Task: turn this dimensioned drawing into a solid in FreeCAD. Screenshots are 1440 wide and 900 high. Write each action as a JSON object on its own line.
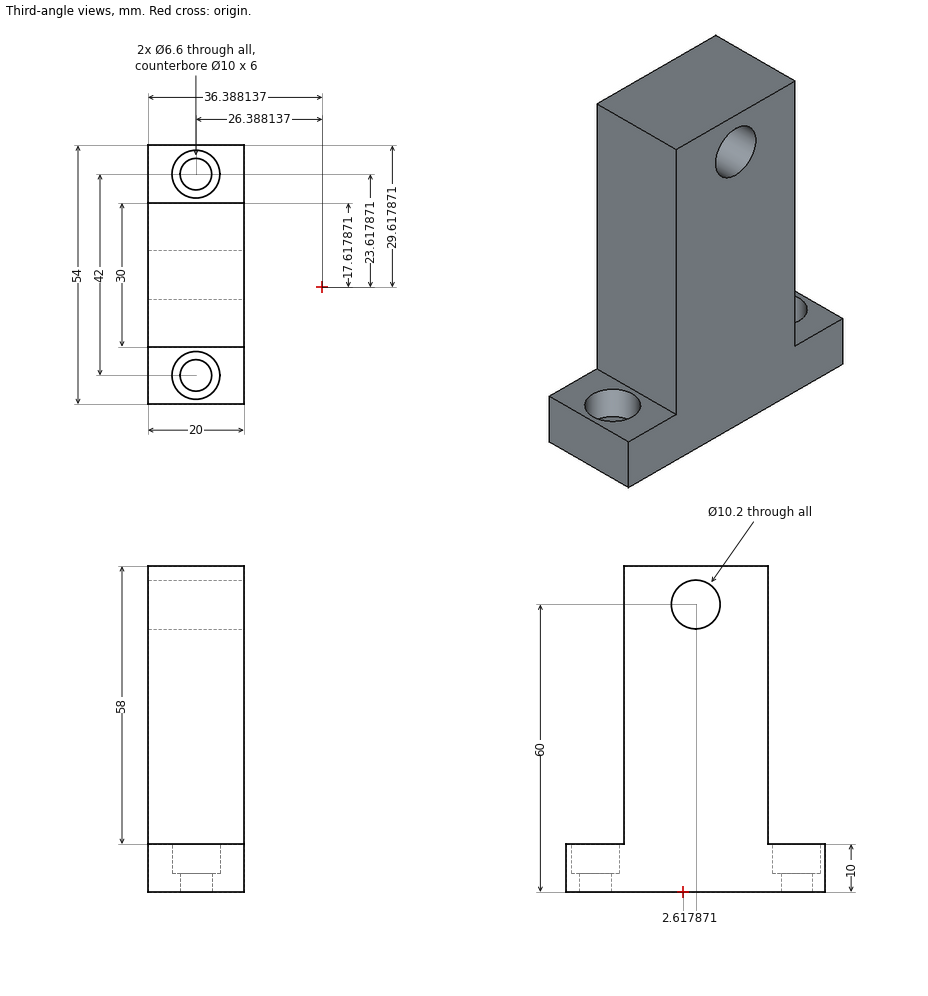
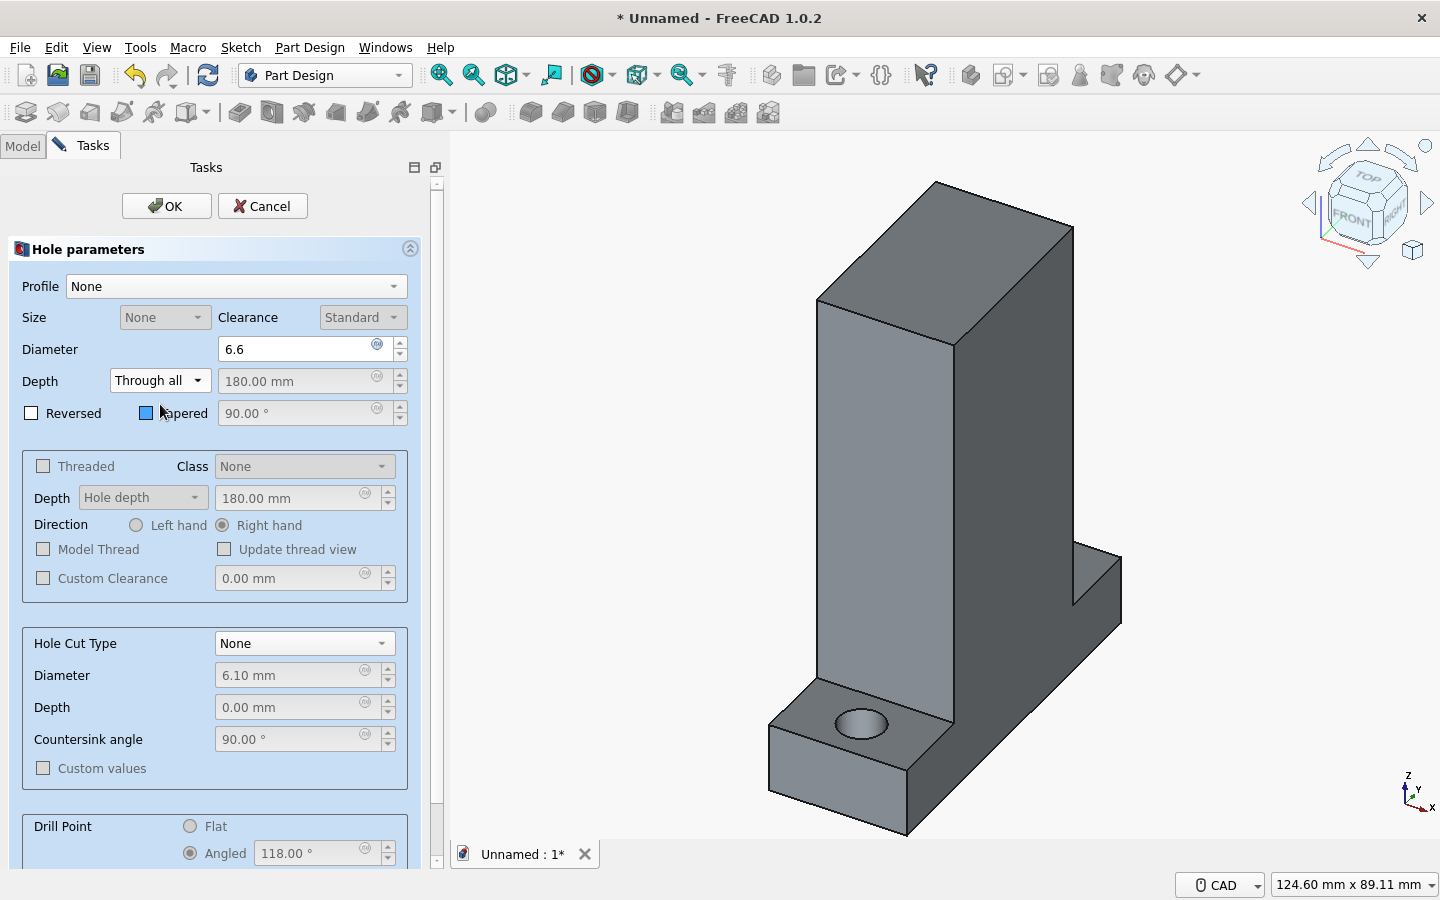
{"action": "left_click", "coordinate": [306, 644]}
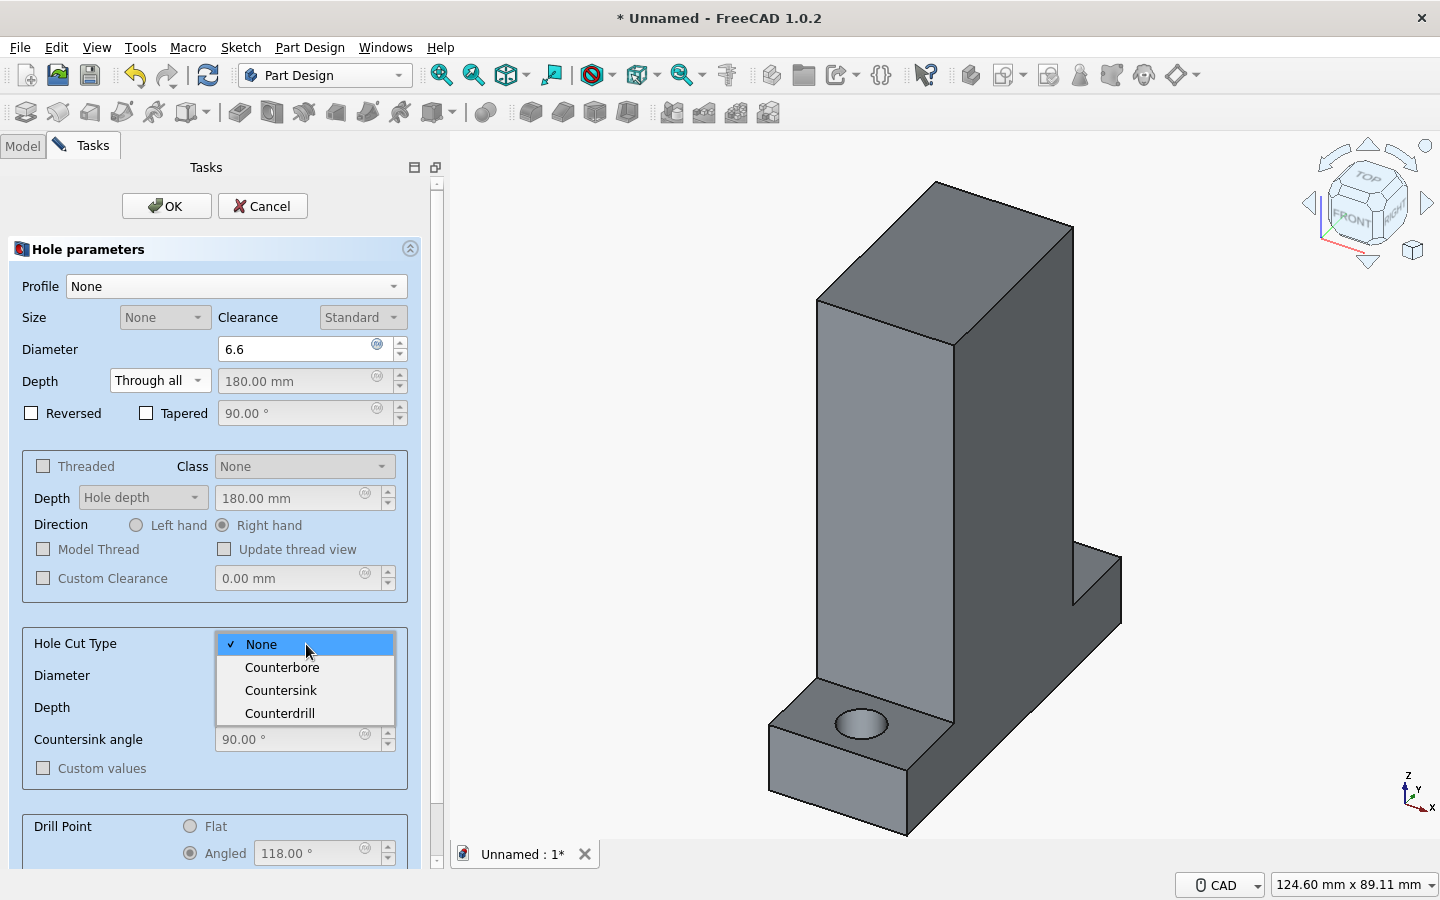
{"action": "left_click", "coordinate": [304, 668]}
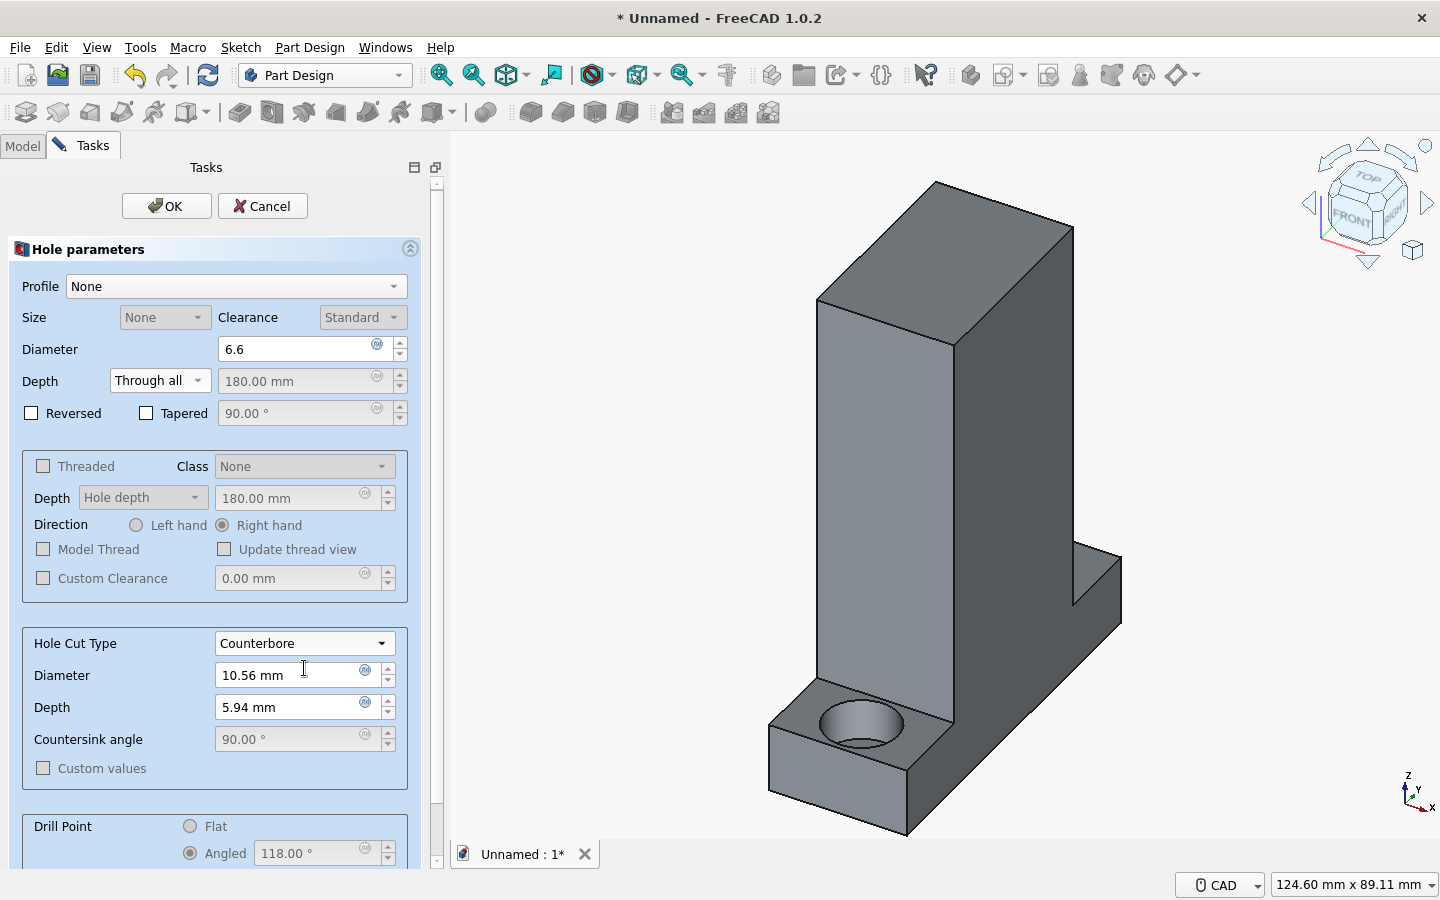
{"action": "triple_click", "coordinate": [298, 675]}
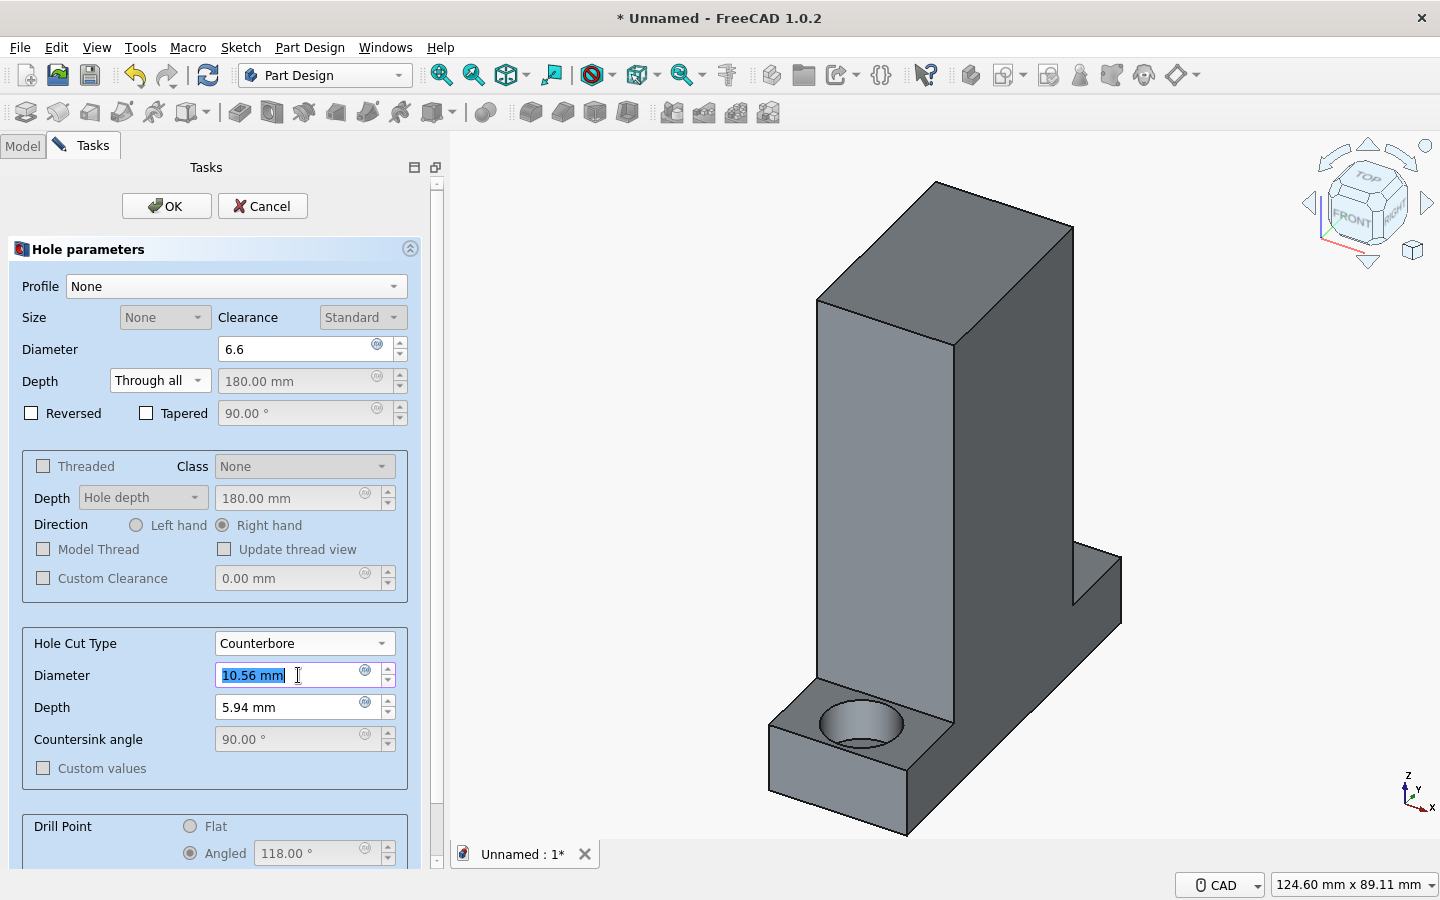
{"action": "type", "text": "10"}
{"action": "key", "text": "Tab"}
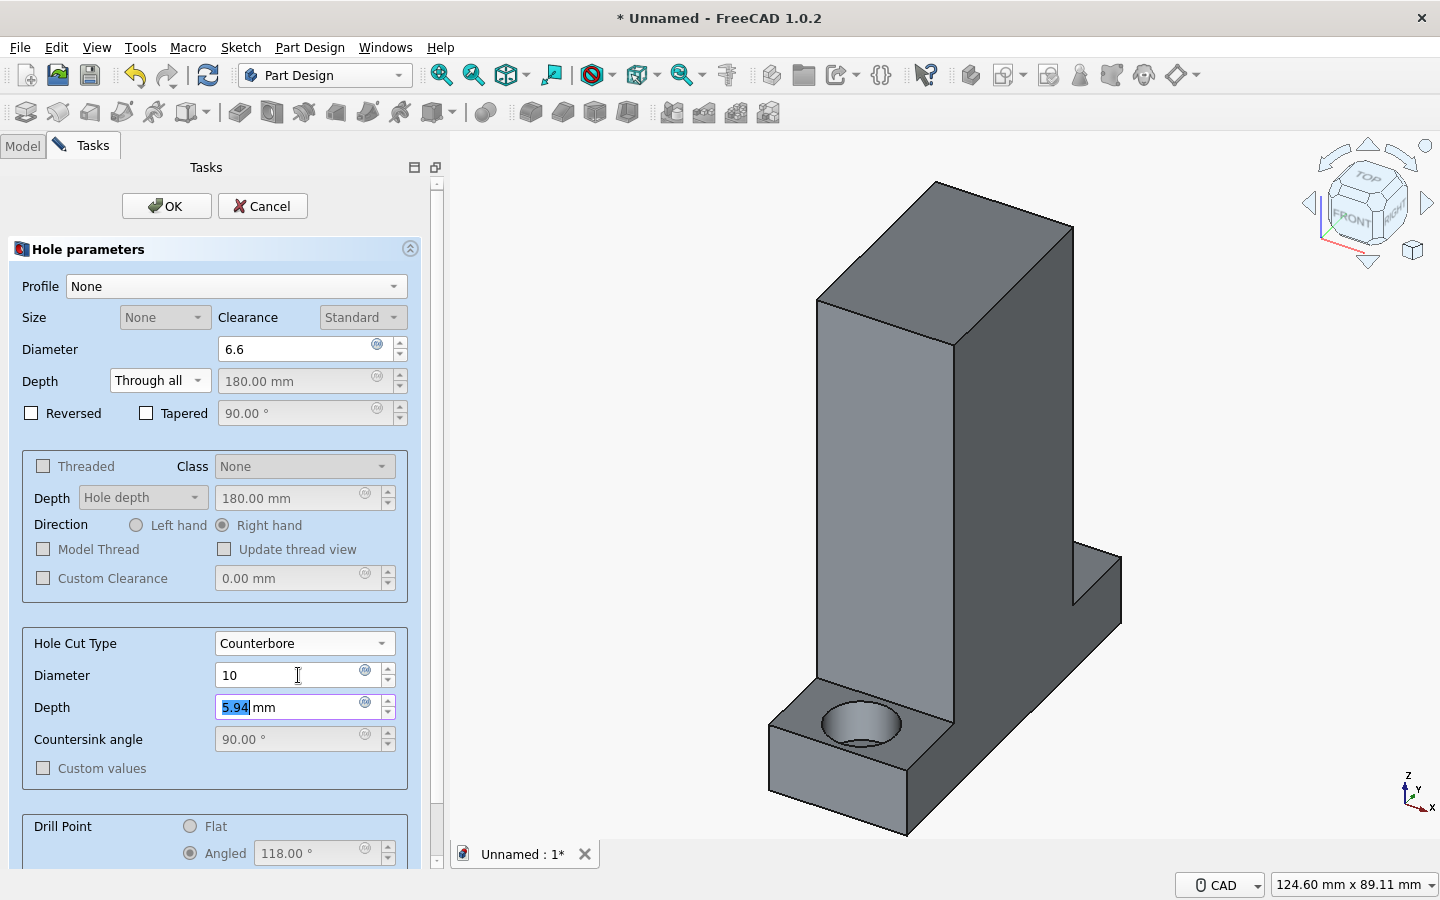
{"action": "type", "text": "6"}
{"action": "key", "text": "Tab"}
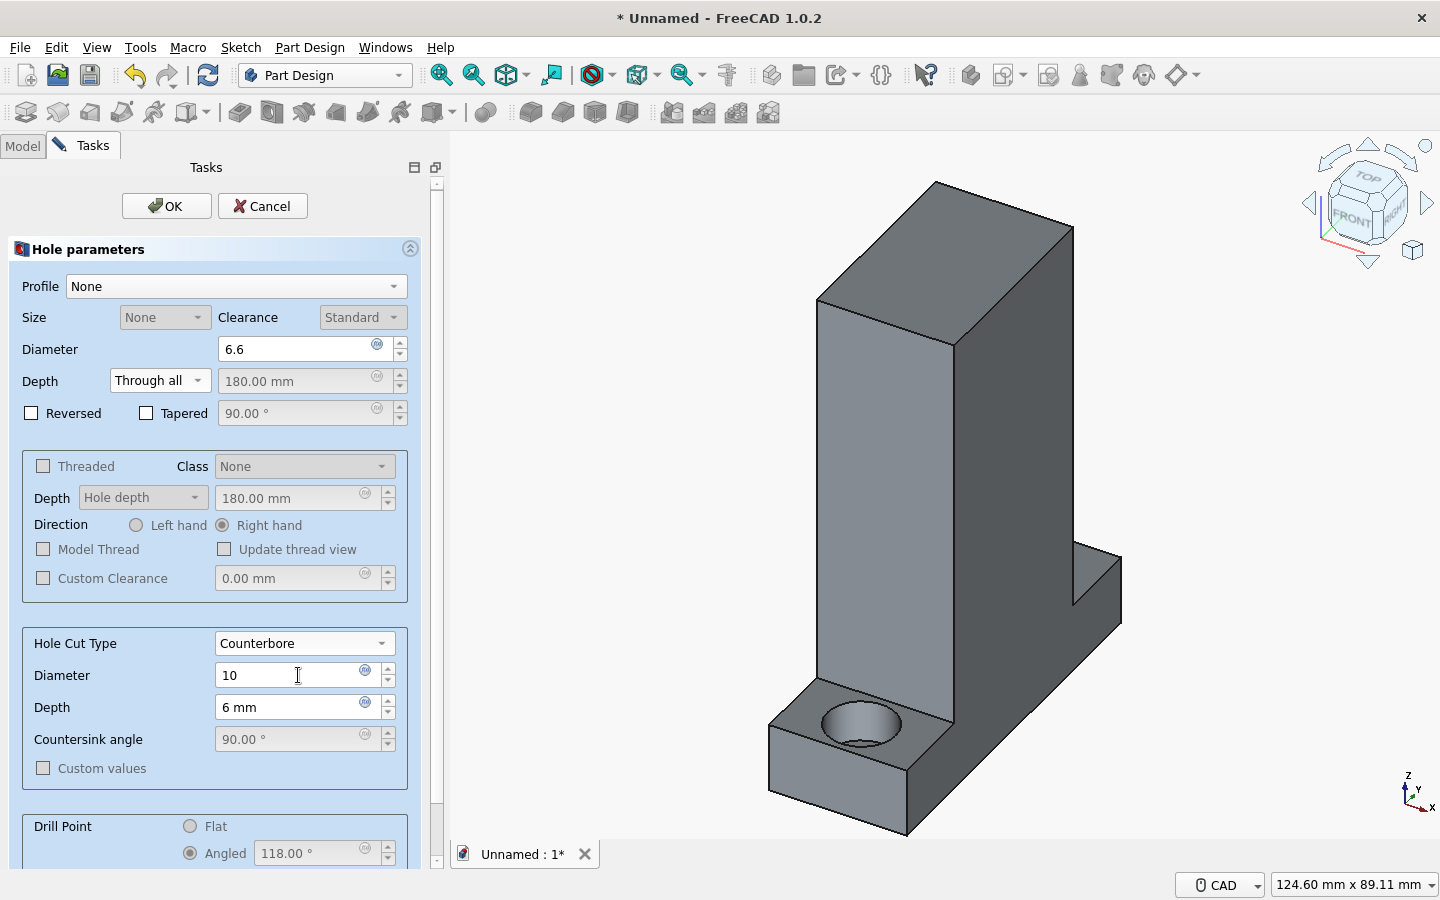
{"action": "left_click", "coordinate": [167, 206]}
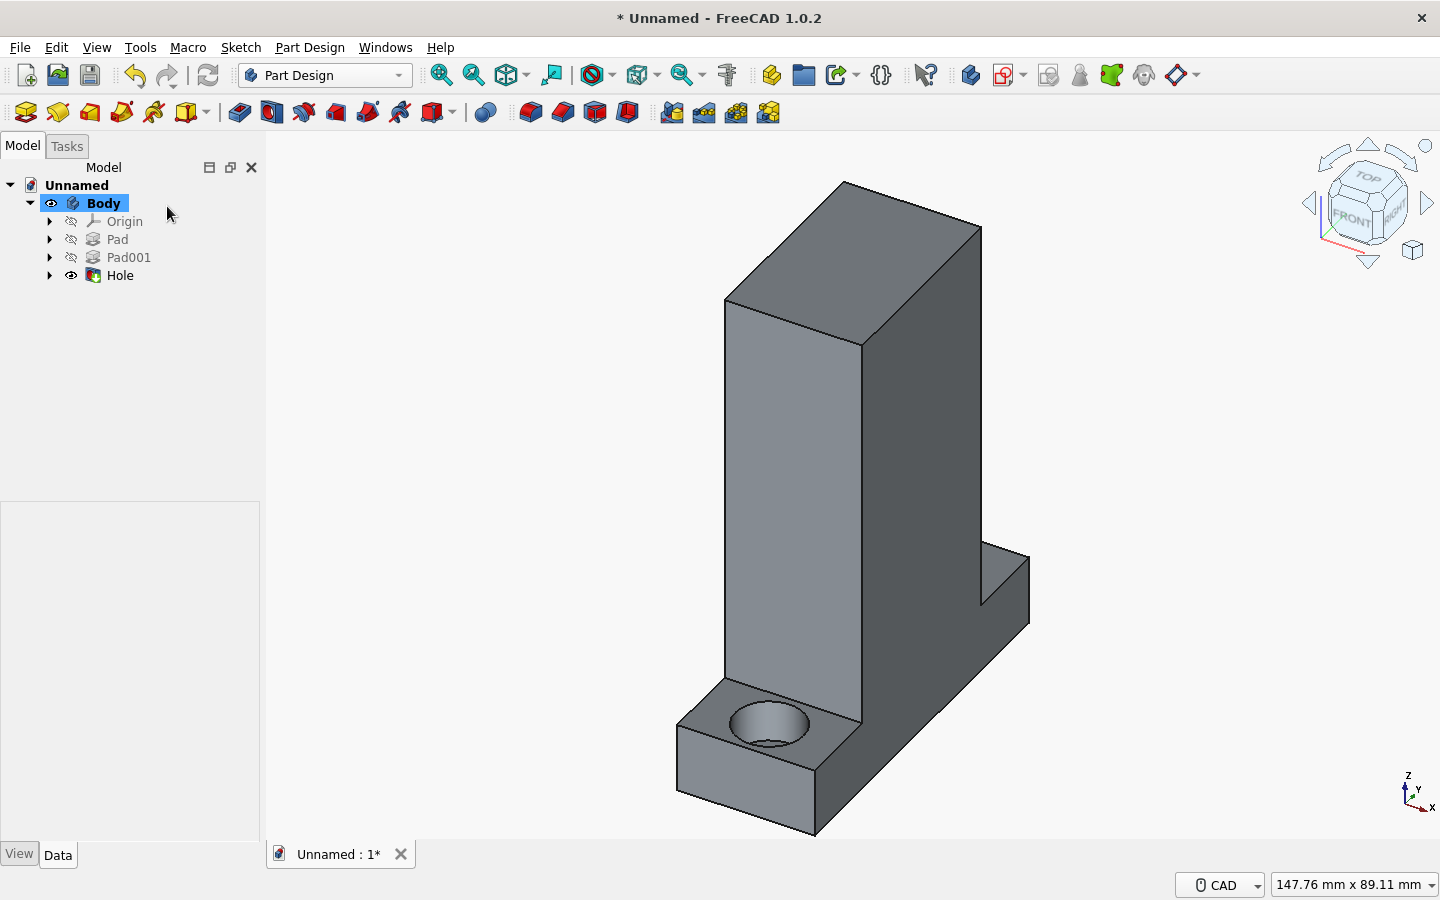
{"action": "key", "text": "6"}